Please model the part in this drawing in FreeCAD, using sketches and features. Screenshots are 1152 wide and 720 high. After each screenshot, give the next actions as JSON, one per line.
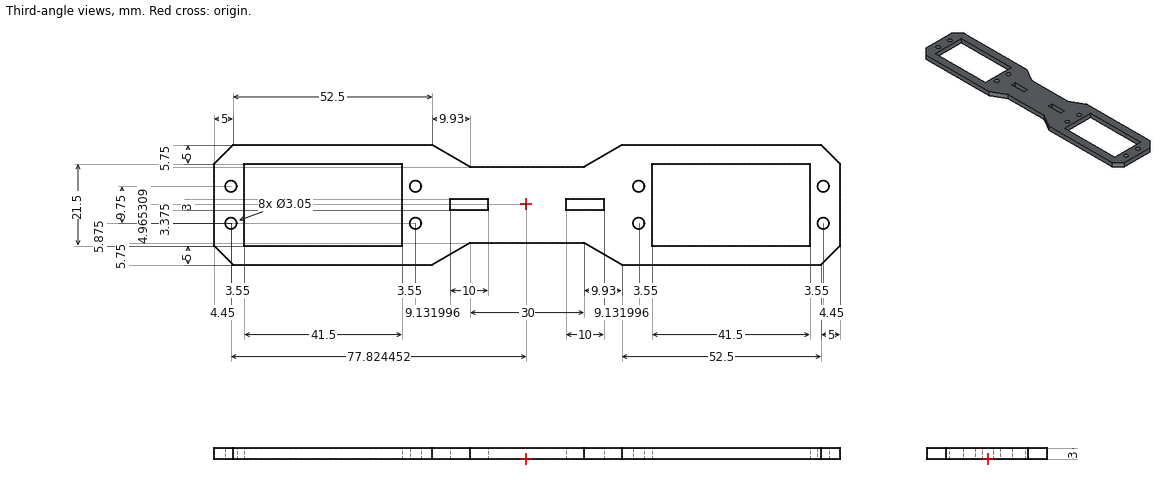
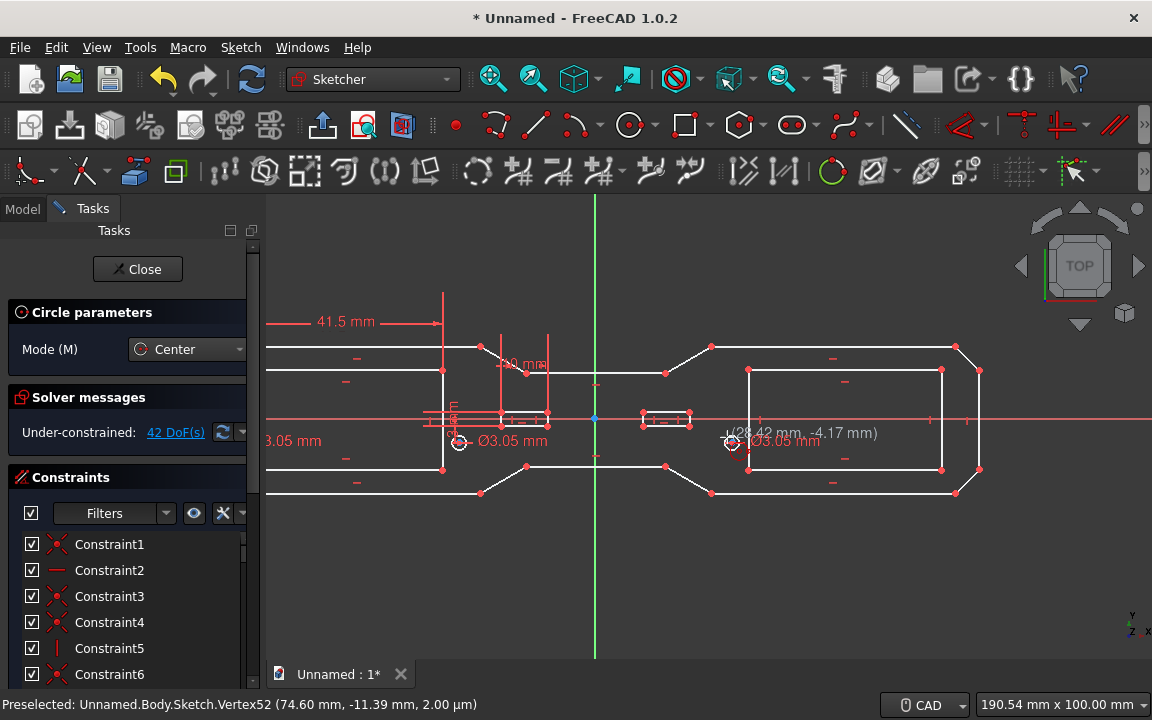
{"action": "scroll", "coordinate": [958, 442], "scroll_direction": "up", "scroll_amount": 6}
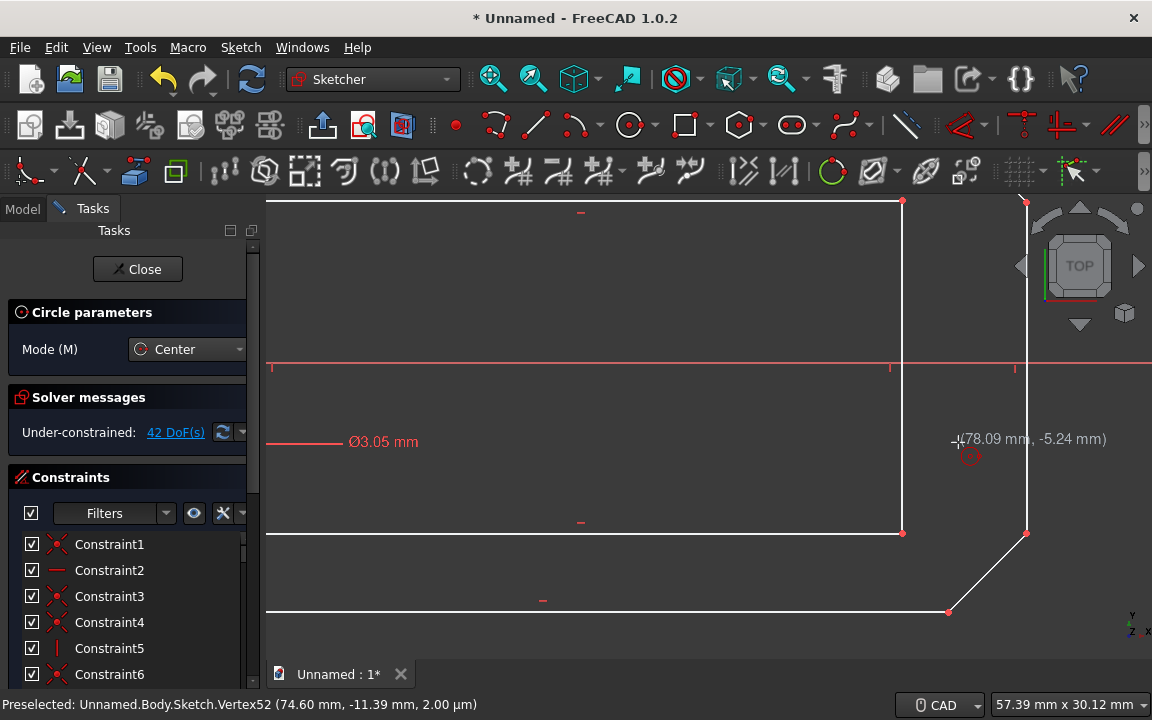
{"action": "scroll", "coordinate": [865, 442], "scroll_direction": "down", "scroll_amount": 8}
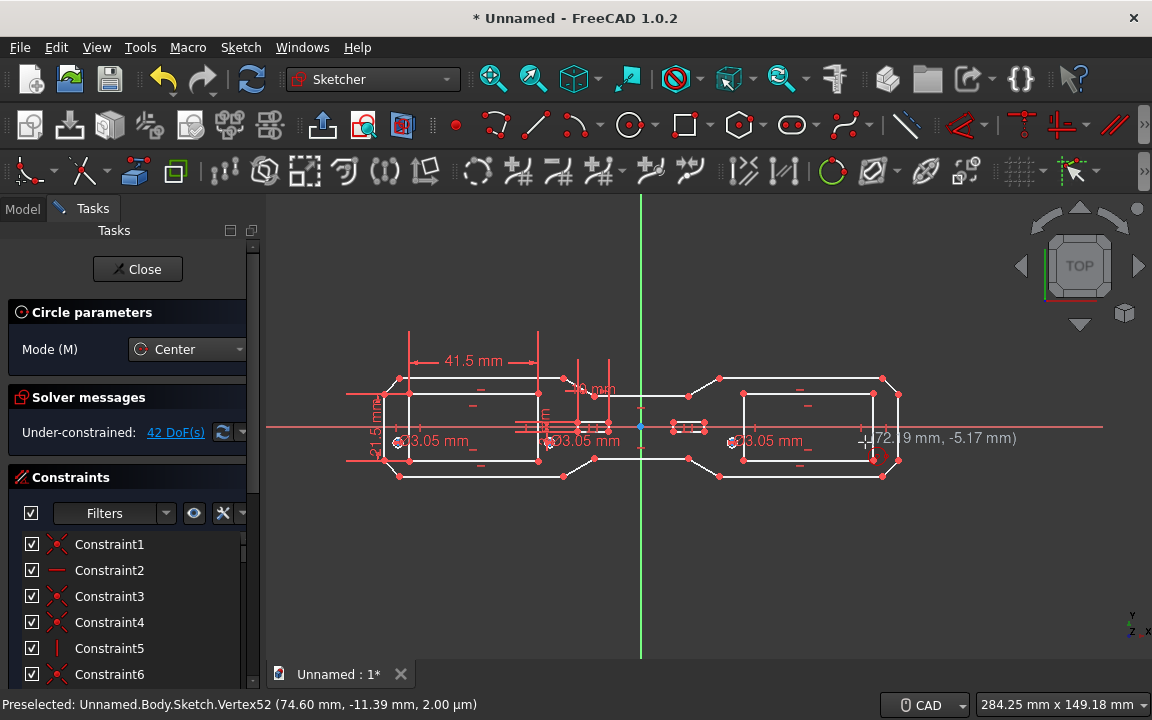
{"action": "scroll", "coordinate": [884, 442], "scroll_direction": "up", "scroll_amount": 2}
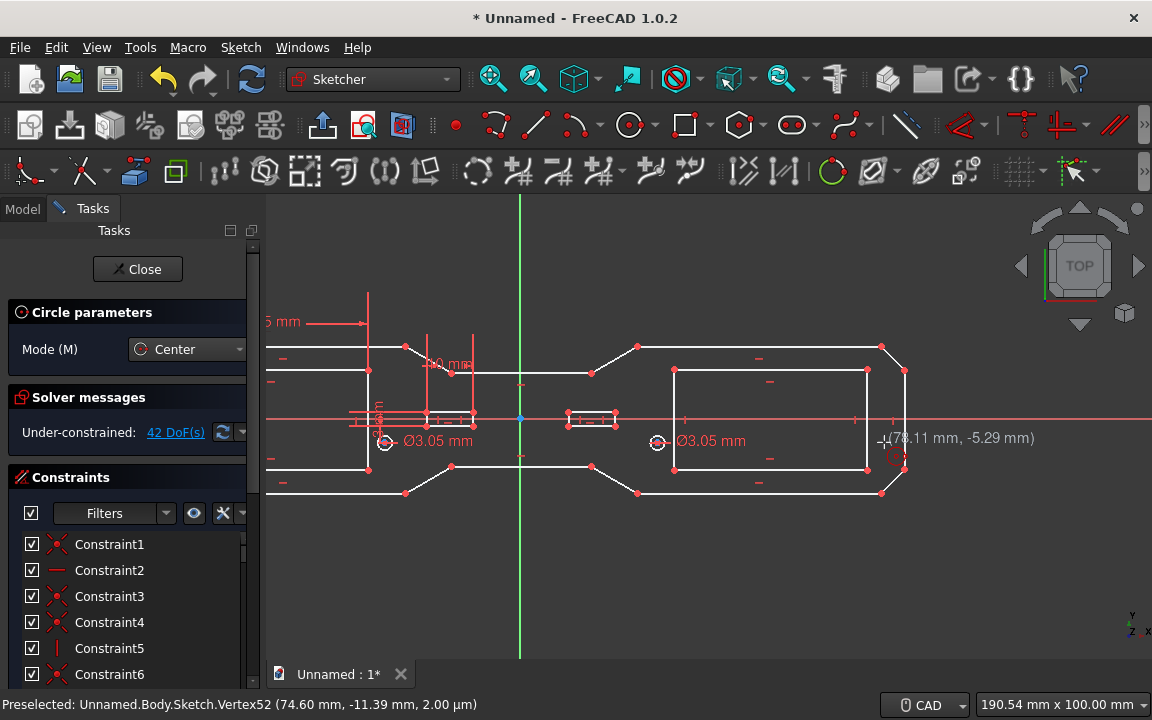
{"action": "left_click", "coordinate": [884, 442]}
{"action": "mouse_move", "coordinate": [889, 437]}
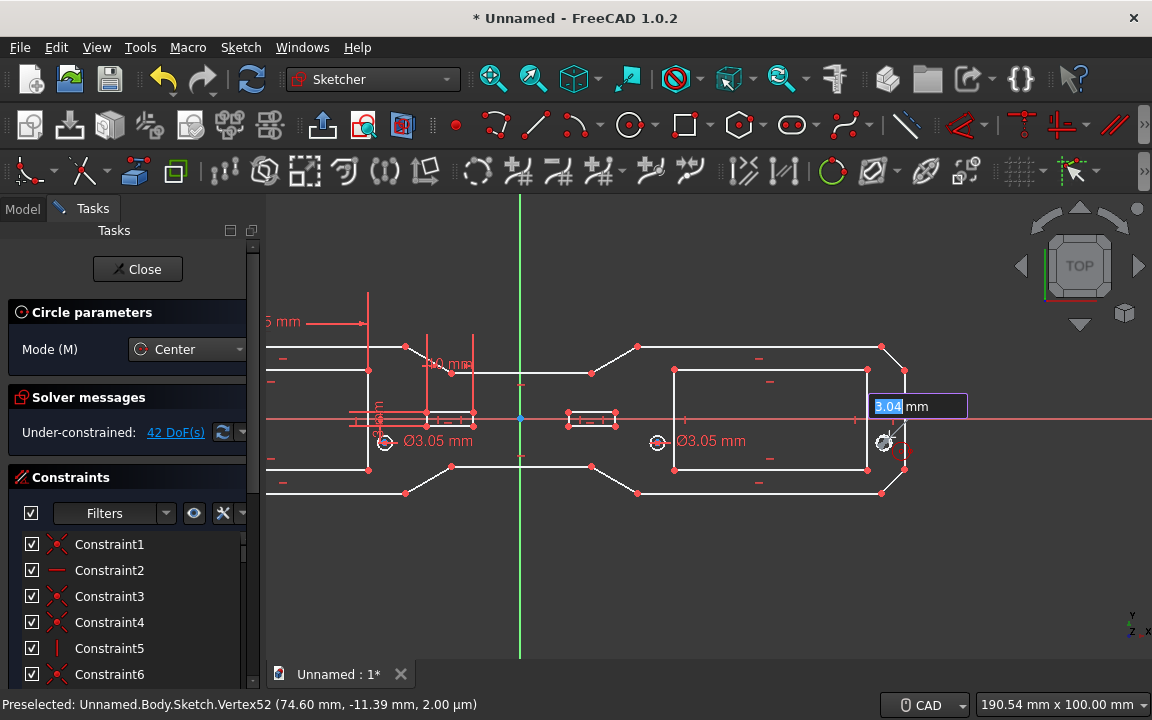
{"action": "type", "text": "3.05"}
{"action": "key", "text": "Return"}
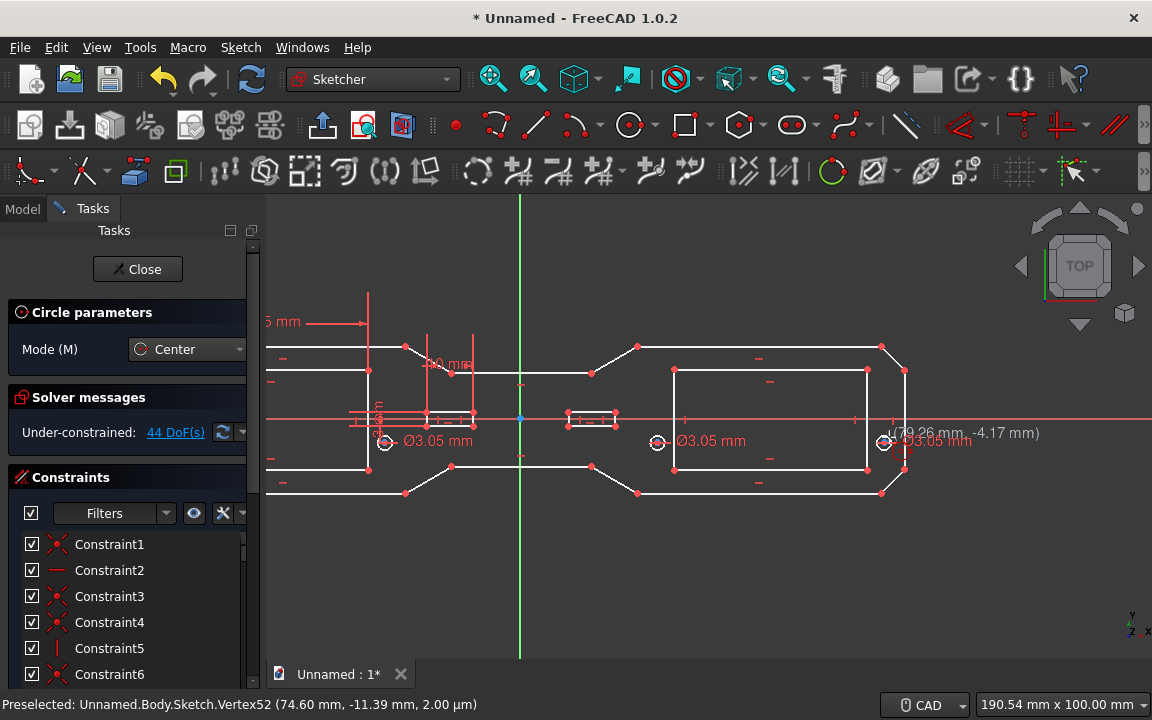
{"action": "scroll", "coordinate": [883, 442], "scroll_direction": "down", "scroll_amount": 2}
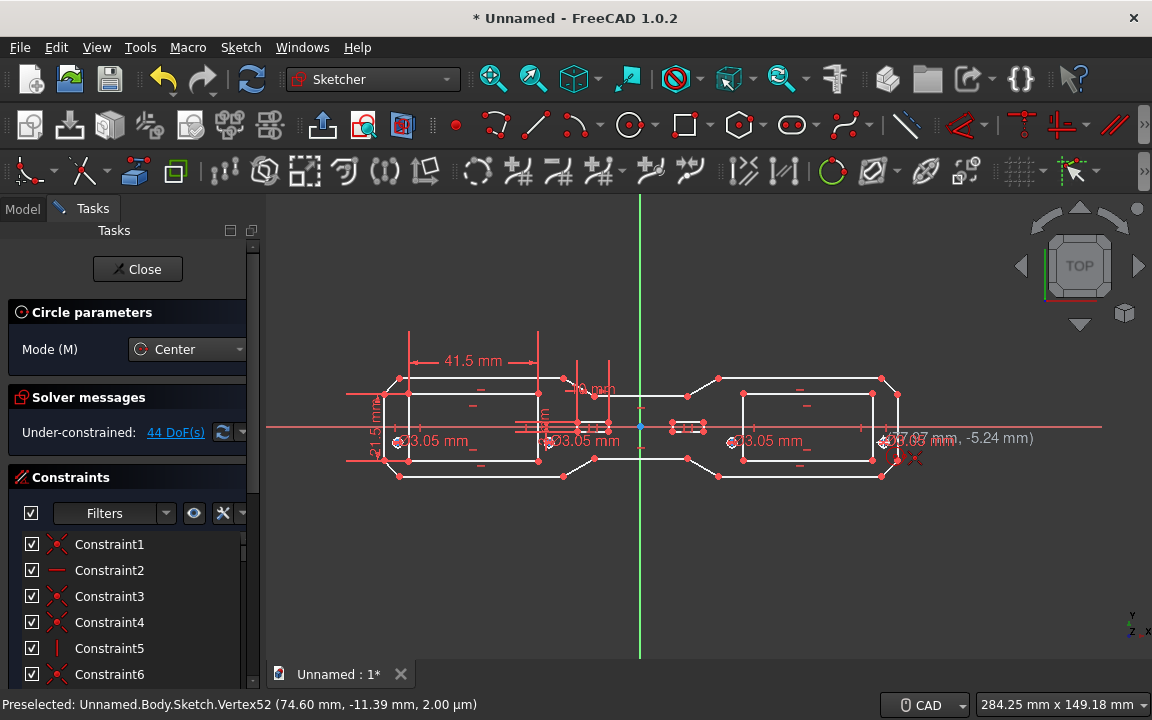
{"action": "scroll", "coordinate": [398, 412], "scroll_direction": "up", "scroll_amount": 8}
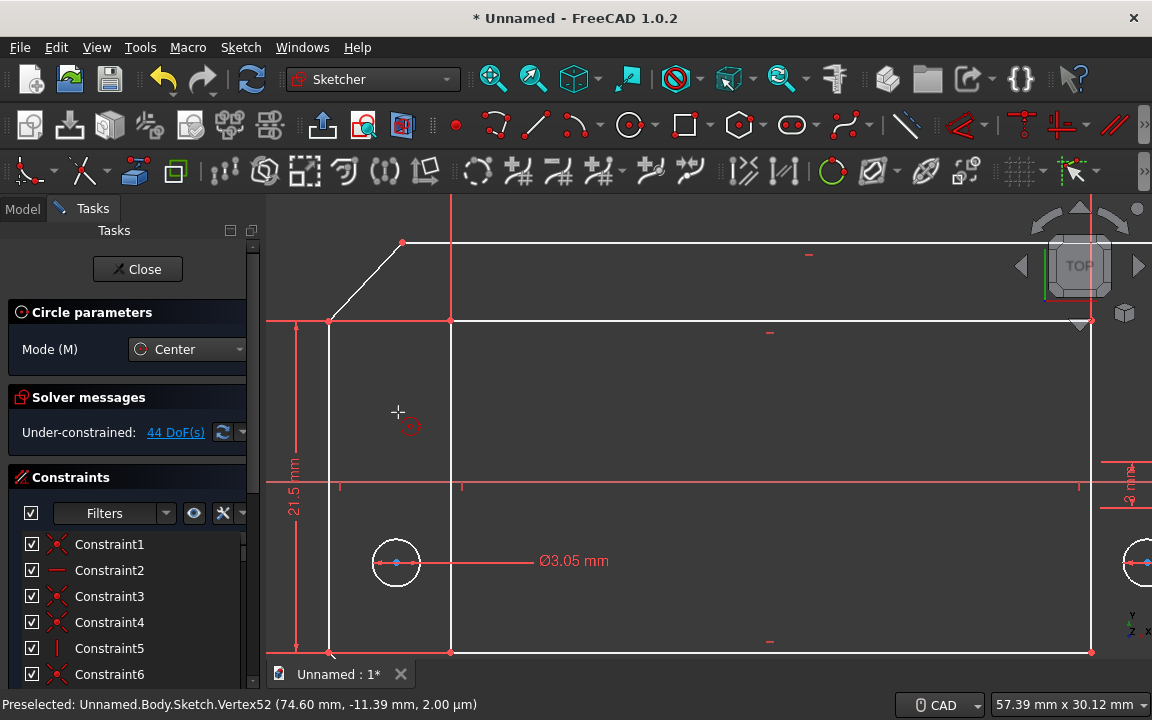
{"action": "scroll", "coordinate": [398, 412], "scroll_direction": "down", "scroll_amount": 8}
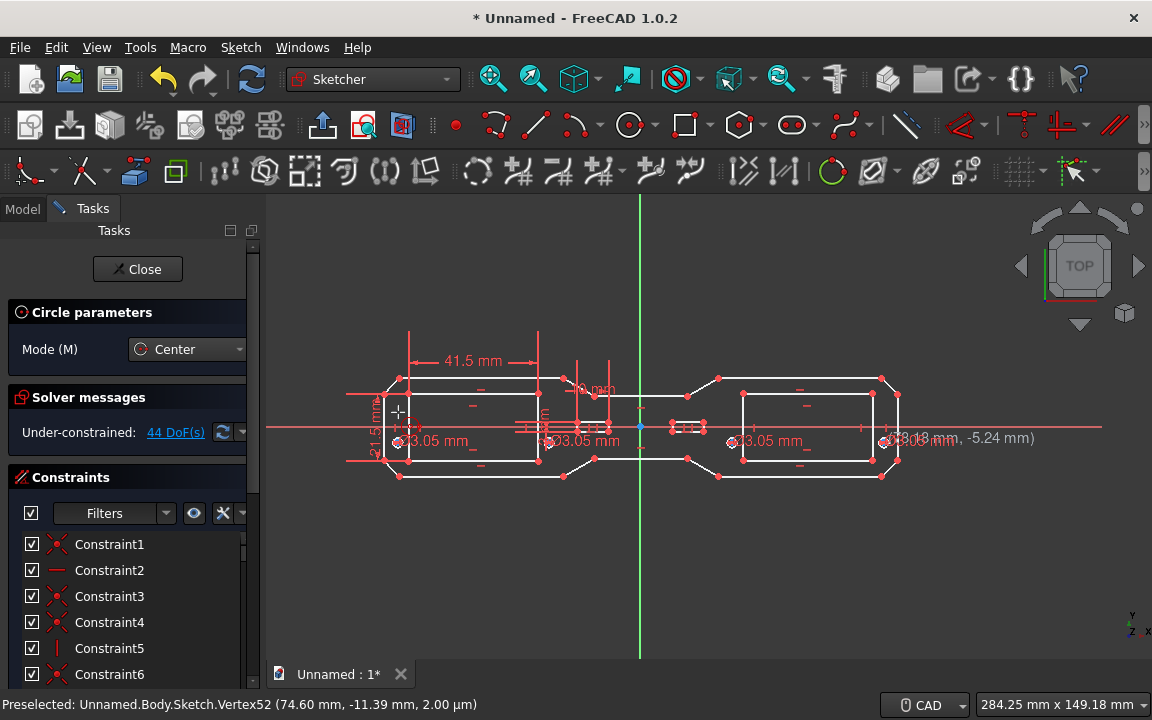
{"action": "scroll", "coordinate": [398, 412], "scroll_direction": "up", "scroll_amount": 2}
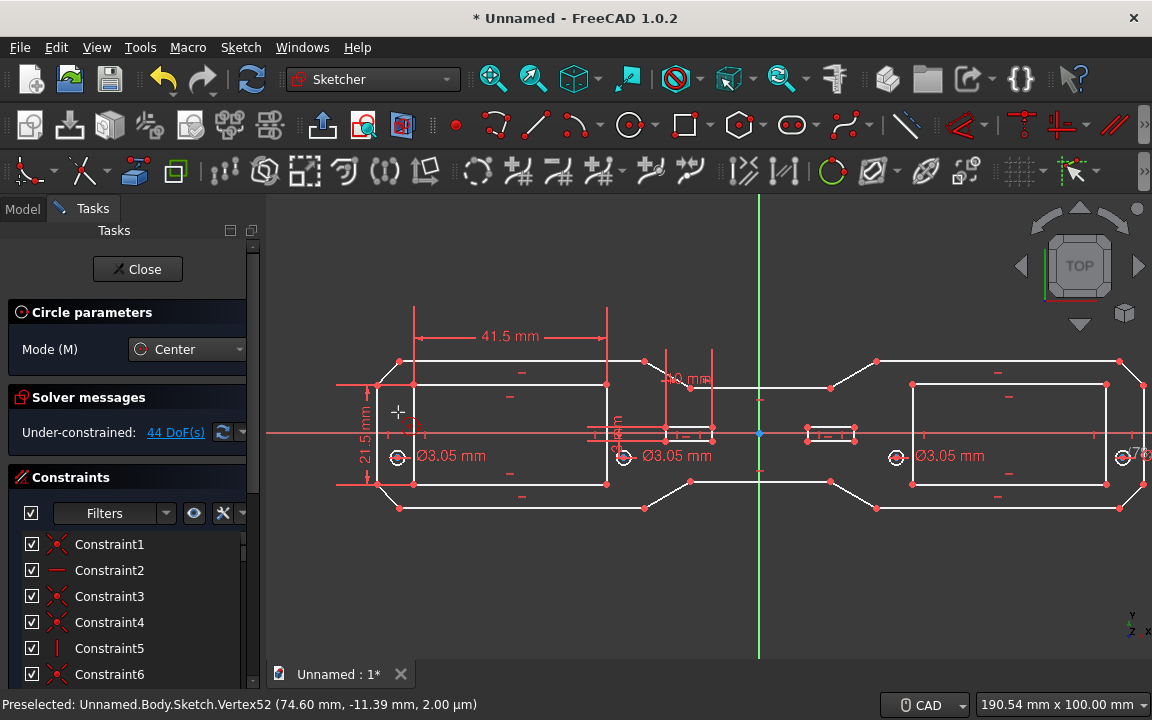
{"action": "left_click", "coordinate": [397, 411]}
{"action": "mouse_move", "coordinate": [392, 406]}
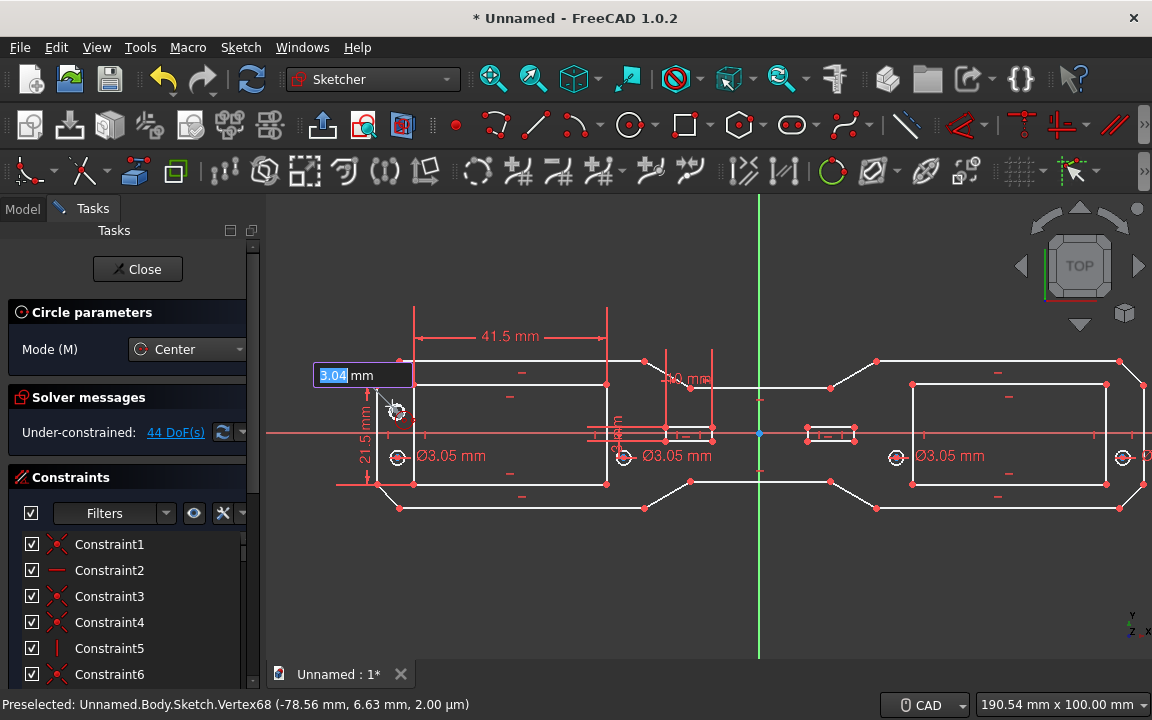
{"action": "type", "text": "3.05"}
{"action": "key", "text": "Return"}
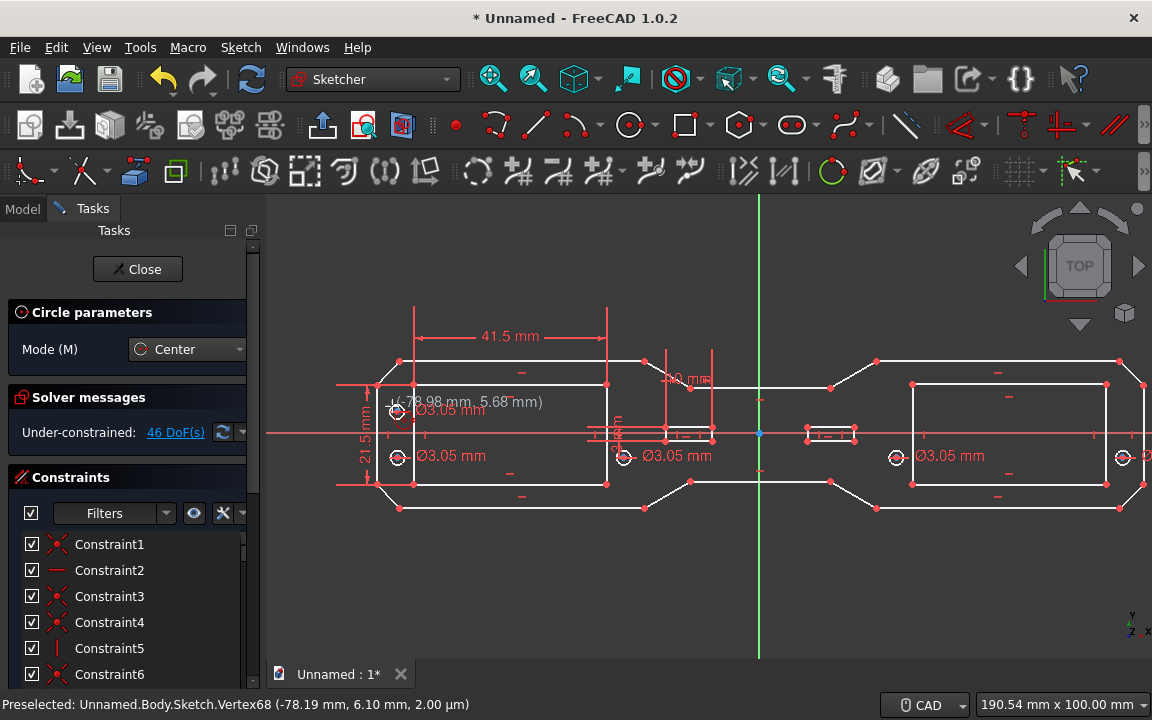
{"action": "scroll", "coordinate": [623, 411], "scroll_direction": "up", "scroll_amount": 6}